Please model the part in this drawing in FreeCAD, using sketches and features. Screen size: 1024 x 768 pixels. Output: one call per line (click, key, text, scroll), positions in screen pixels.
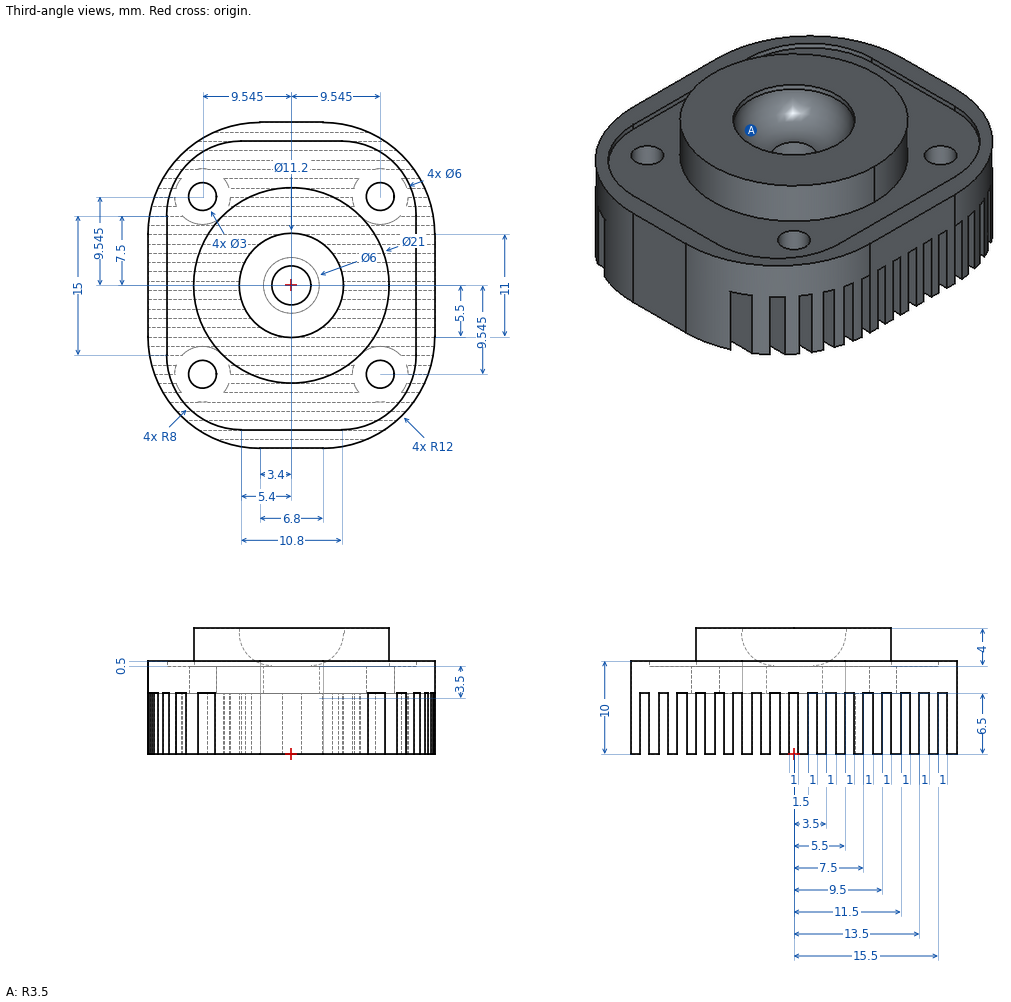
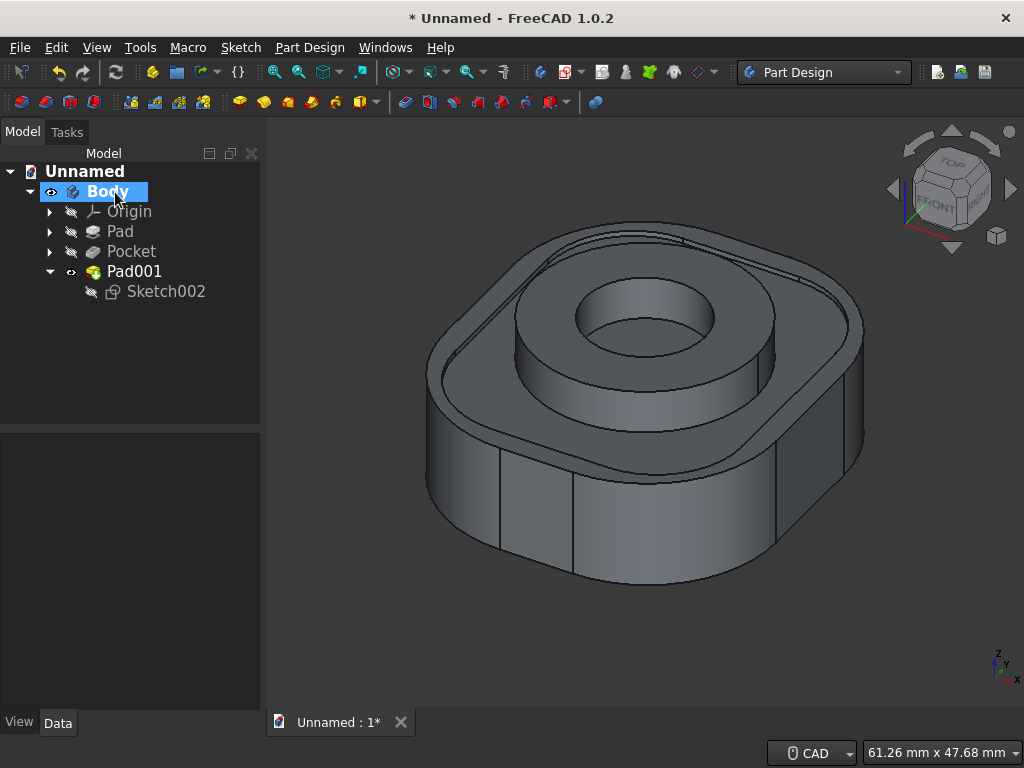
key(0)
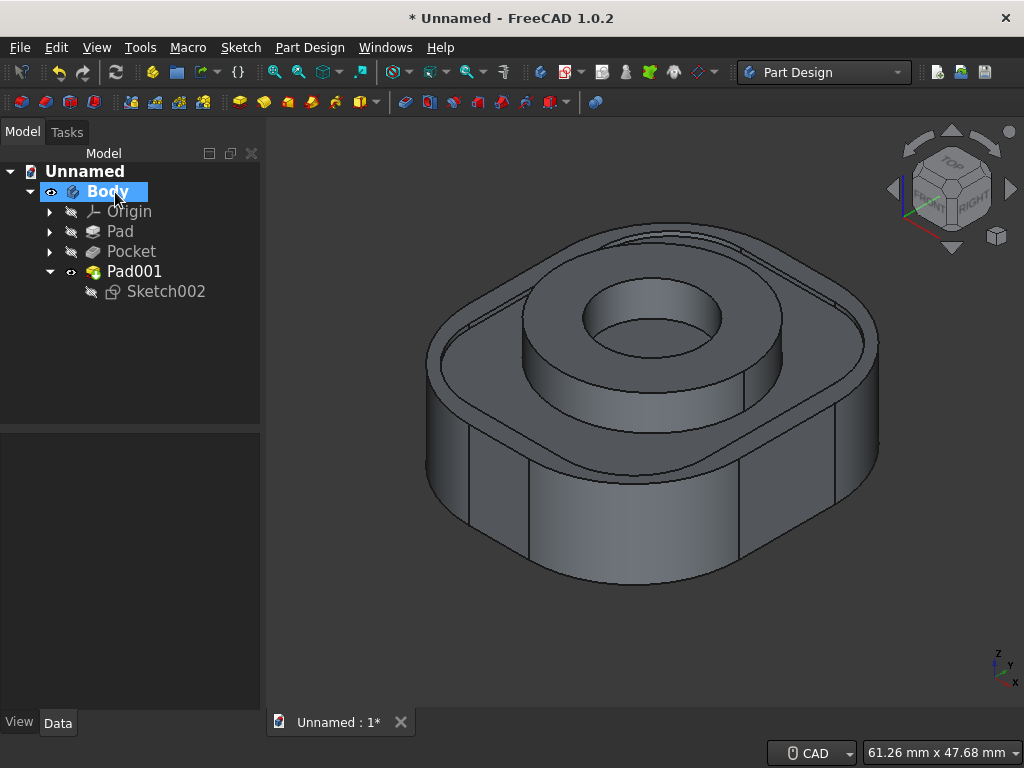
key(2)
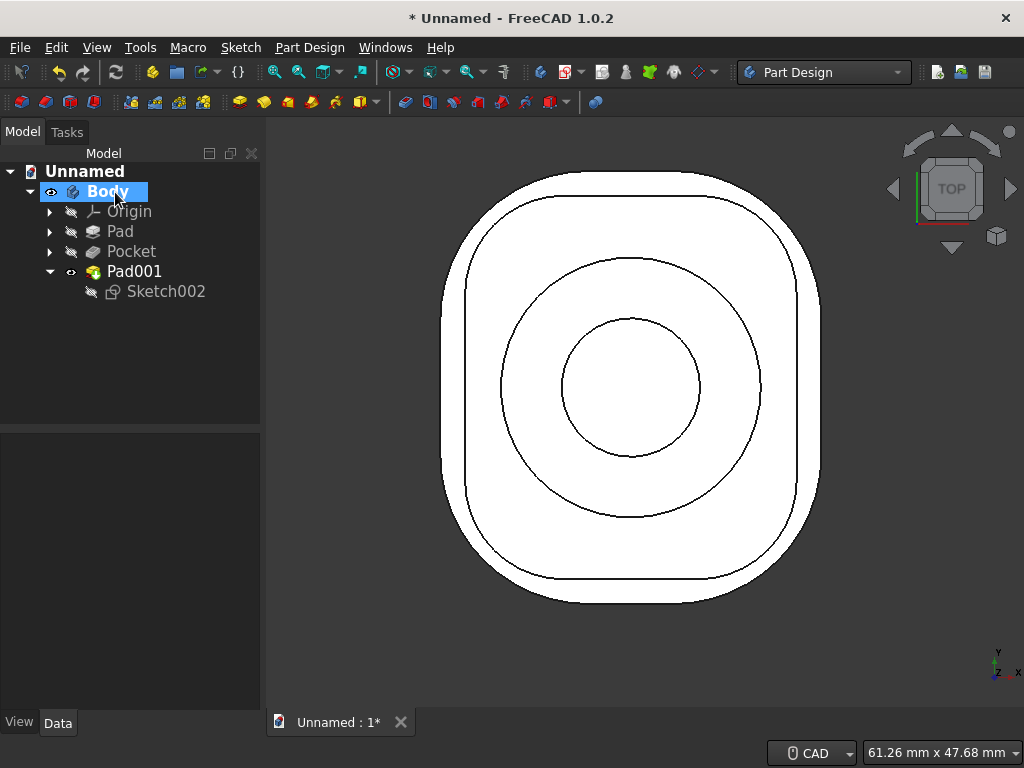
key(1)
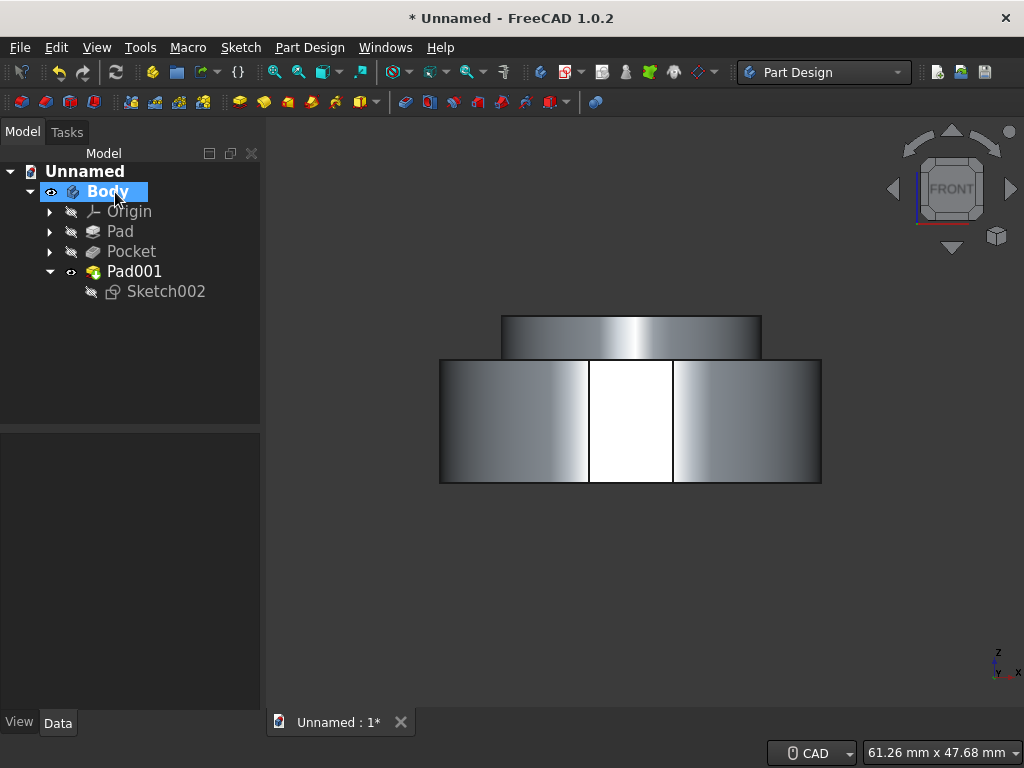
key(3)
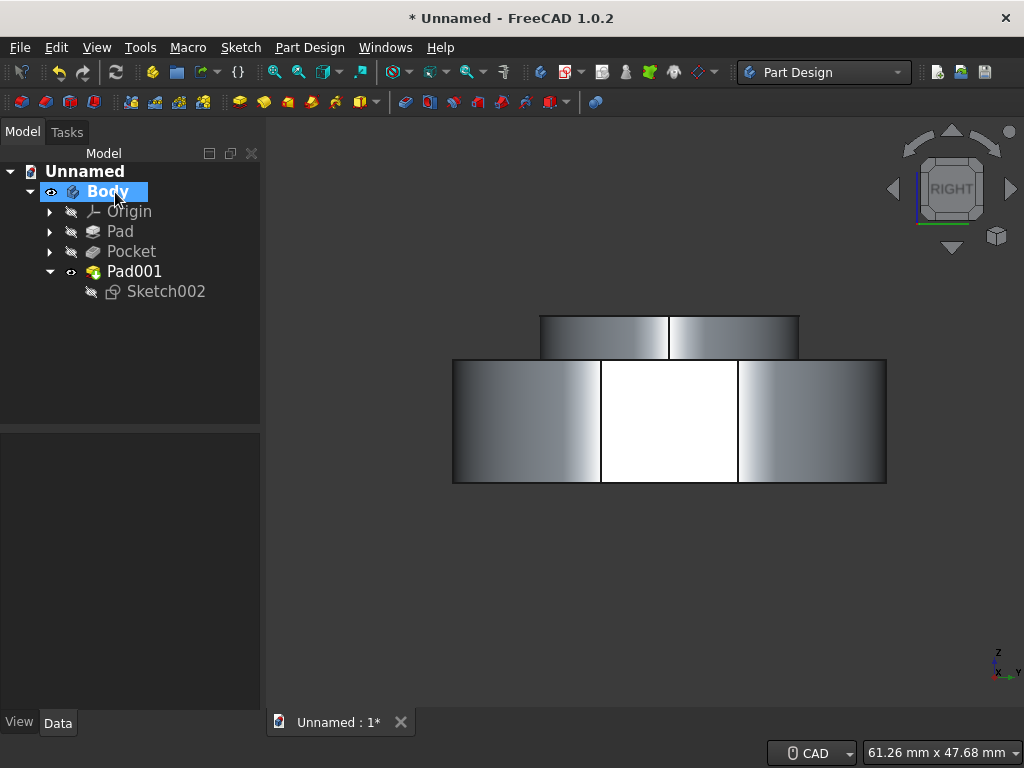
key(5)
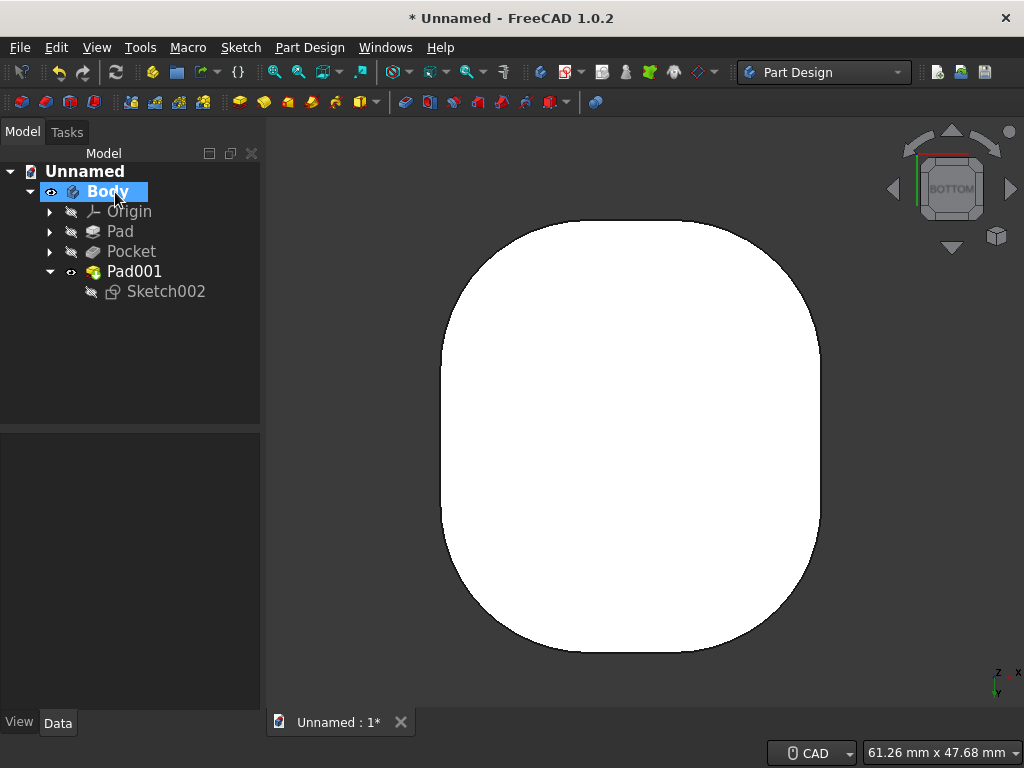
key(4)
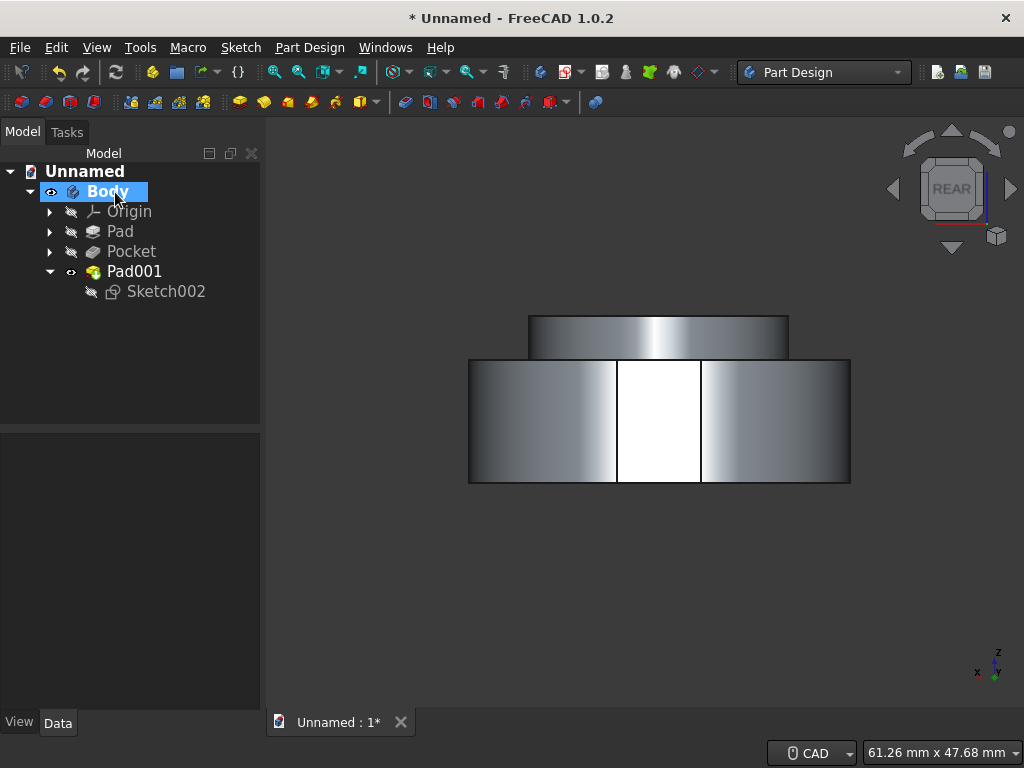
key(6)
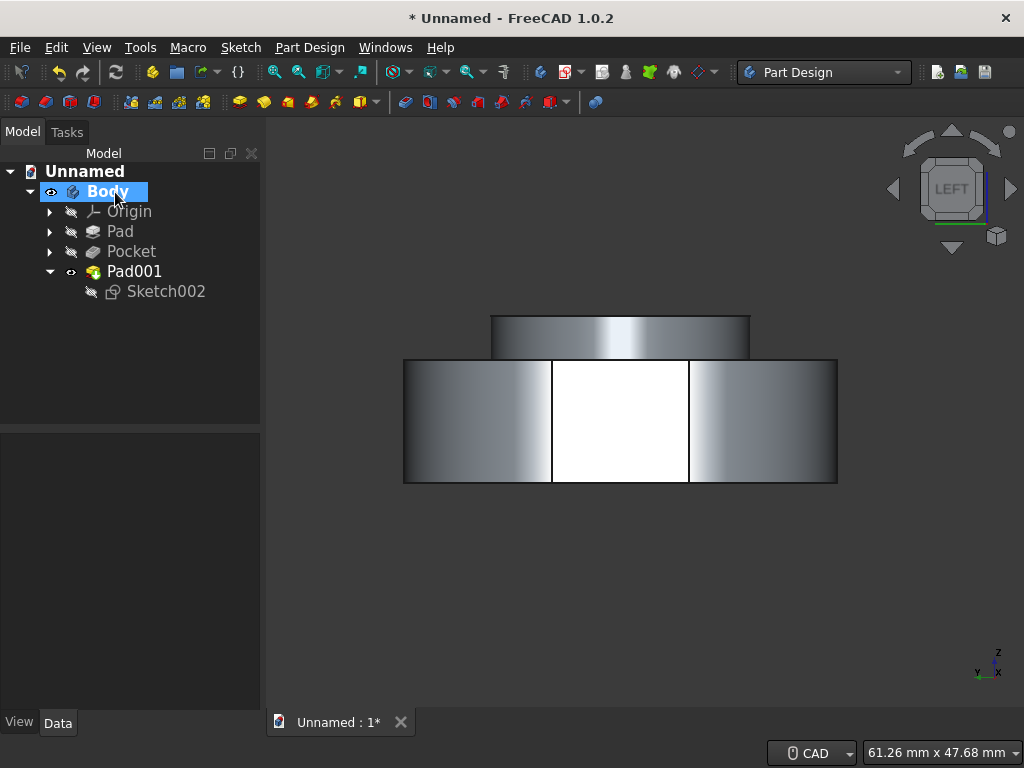
key(v)
key(3)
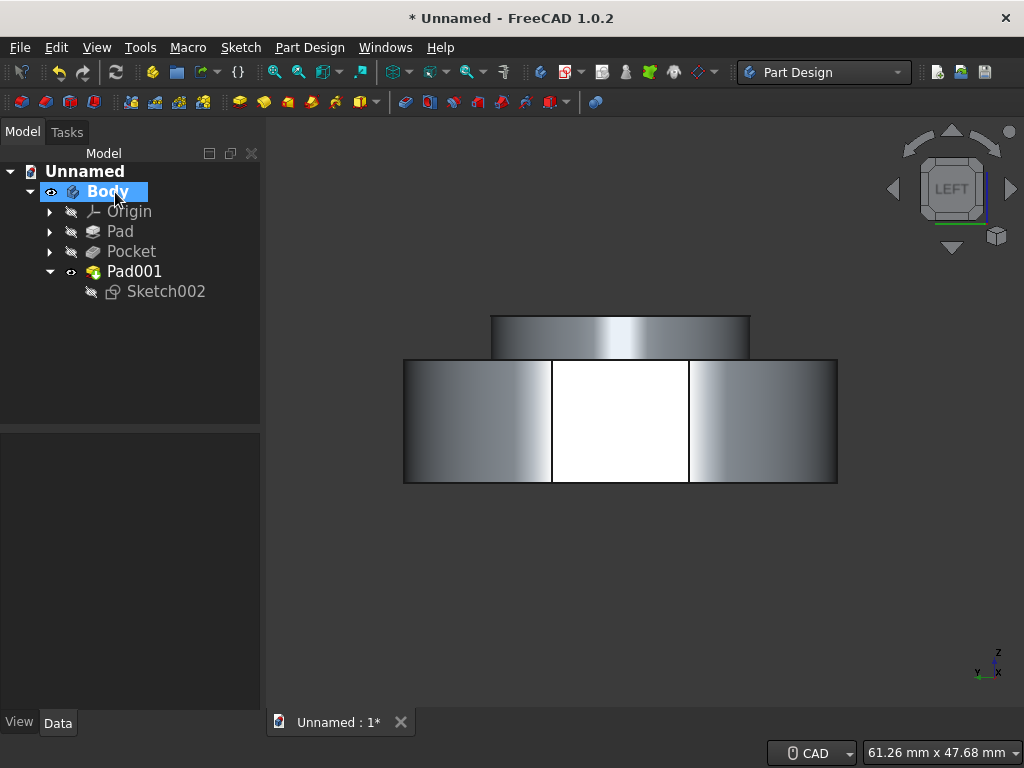
key(0)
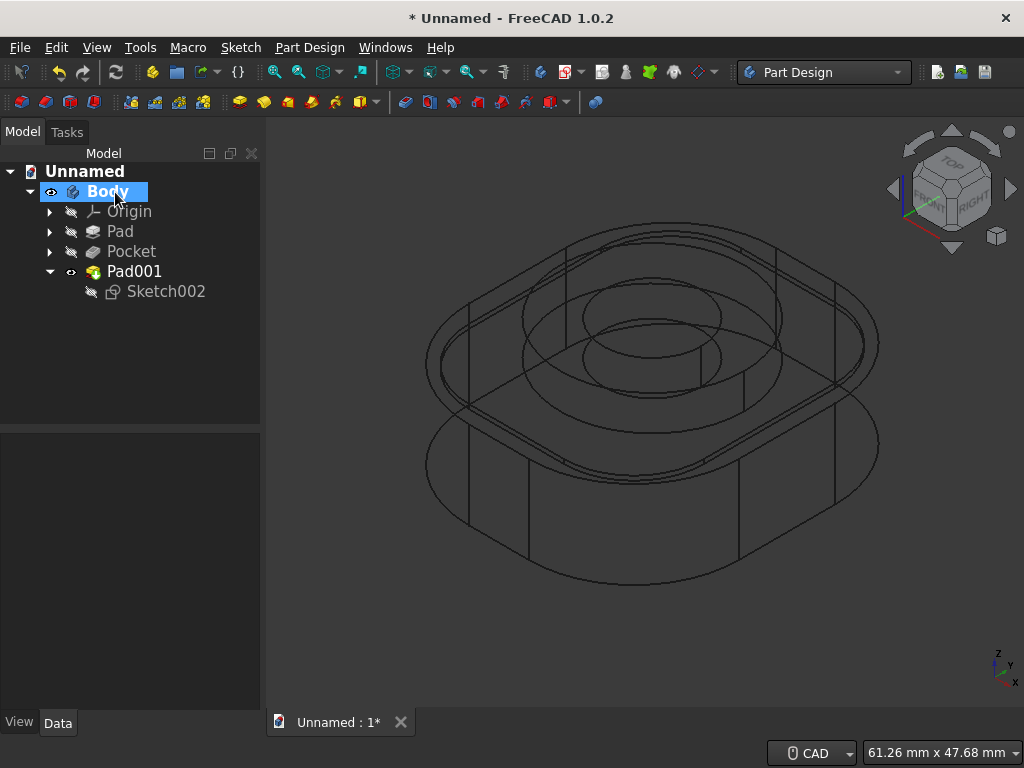
click(603, 329)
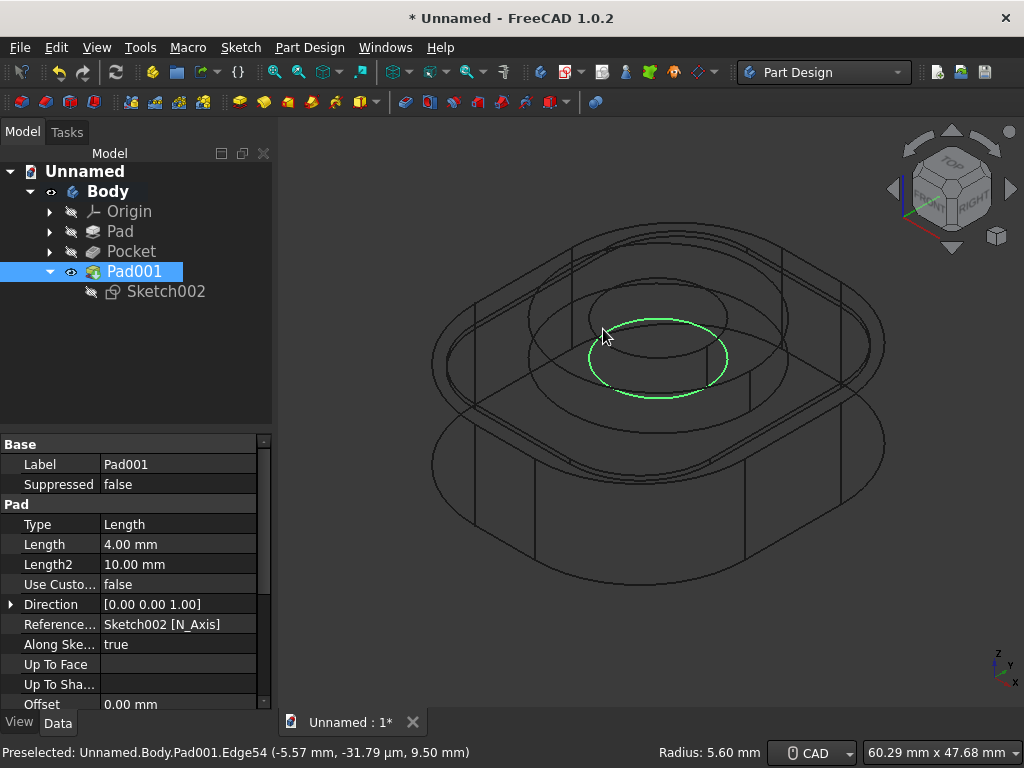
key(v)
key(1)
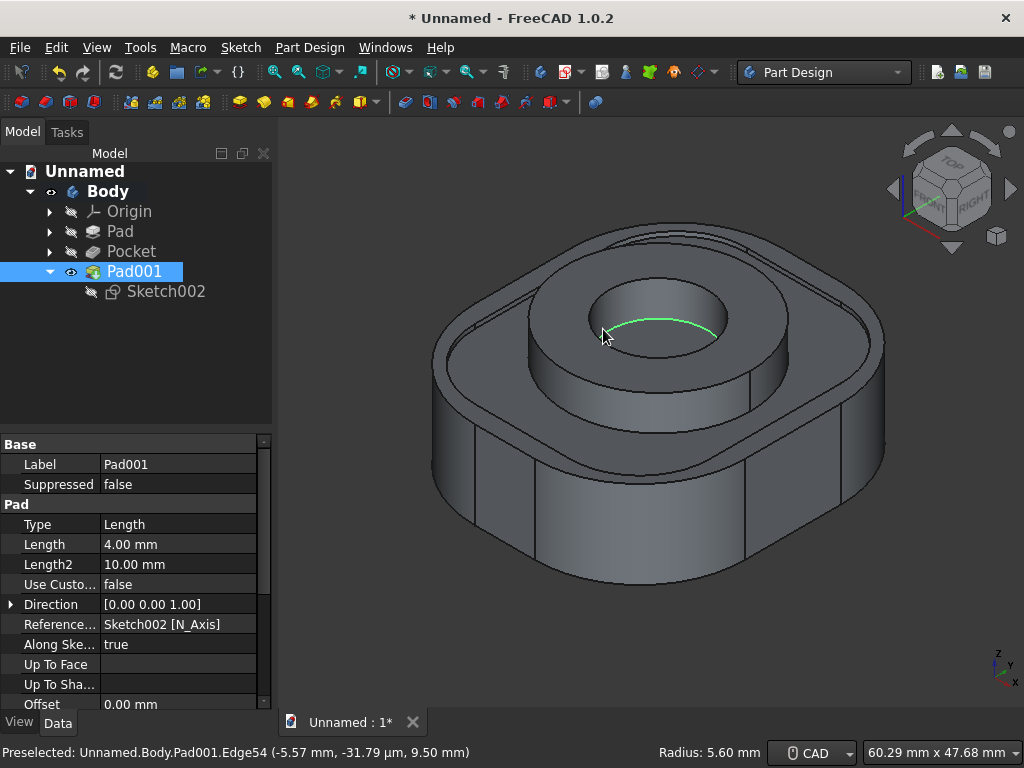
click(22, 102)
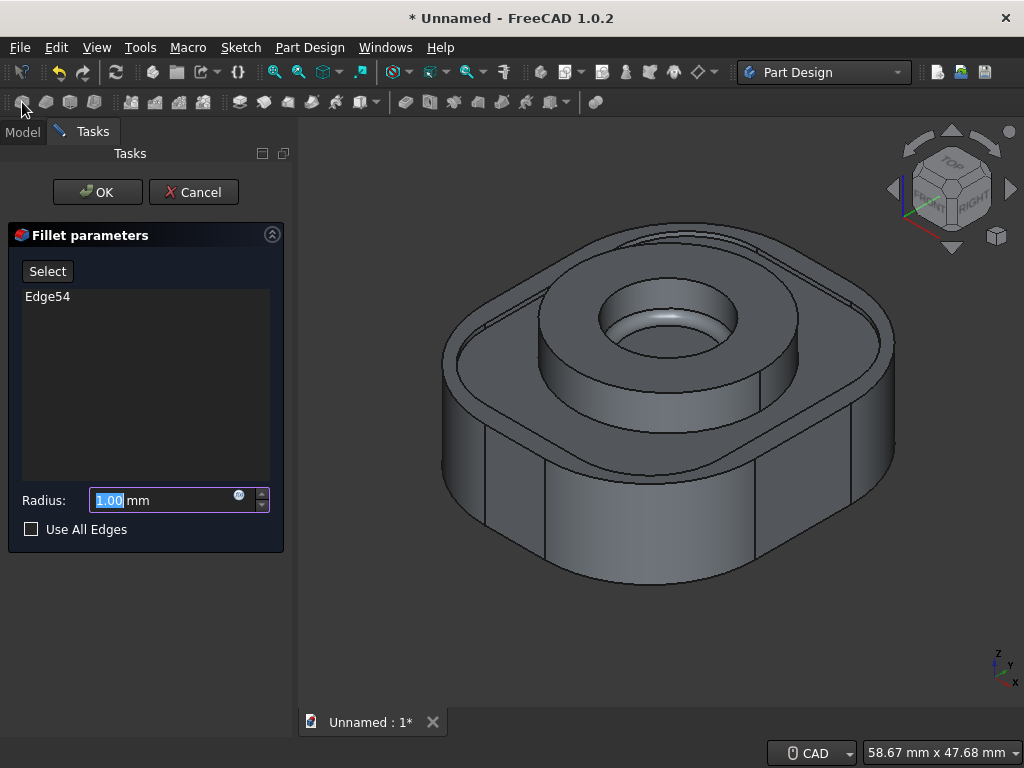
text(3.5)
key(Tab)